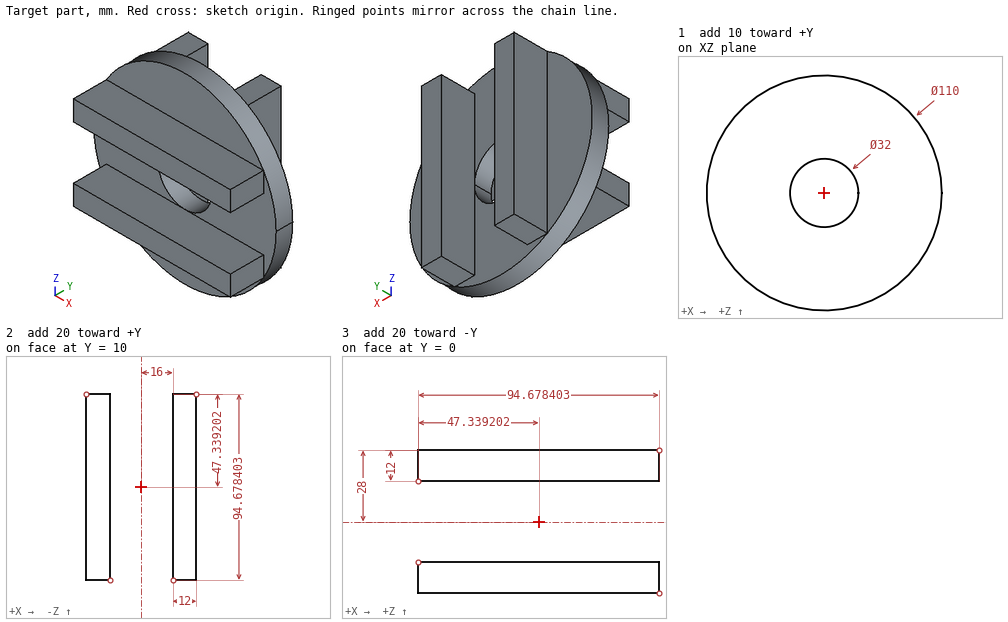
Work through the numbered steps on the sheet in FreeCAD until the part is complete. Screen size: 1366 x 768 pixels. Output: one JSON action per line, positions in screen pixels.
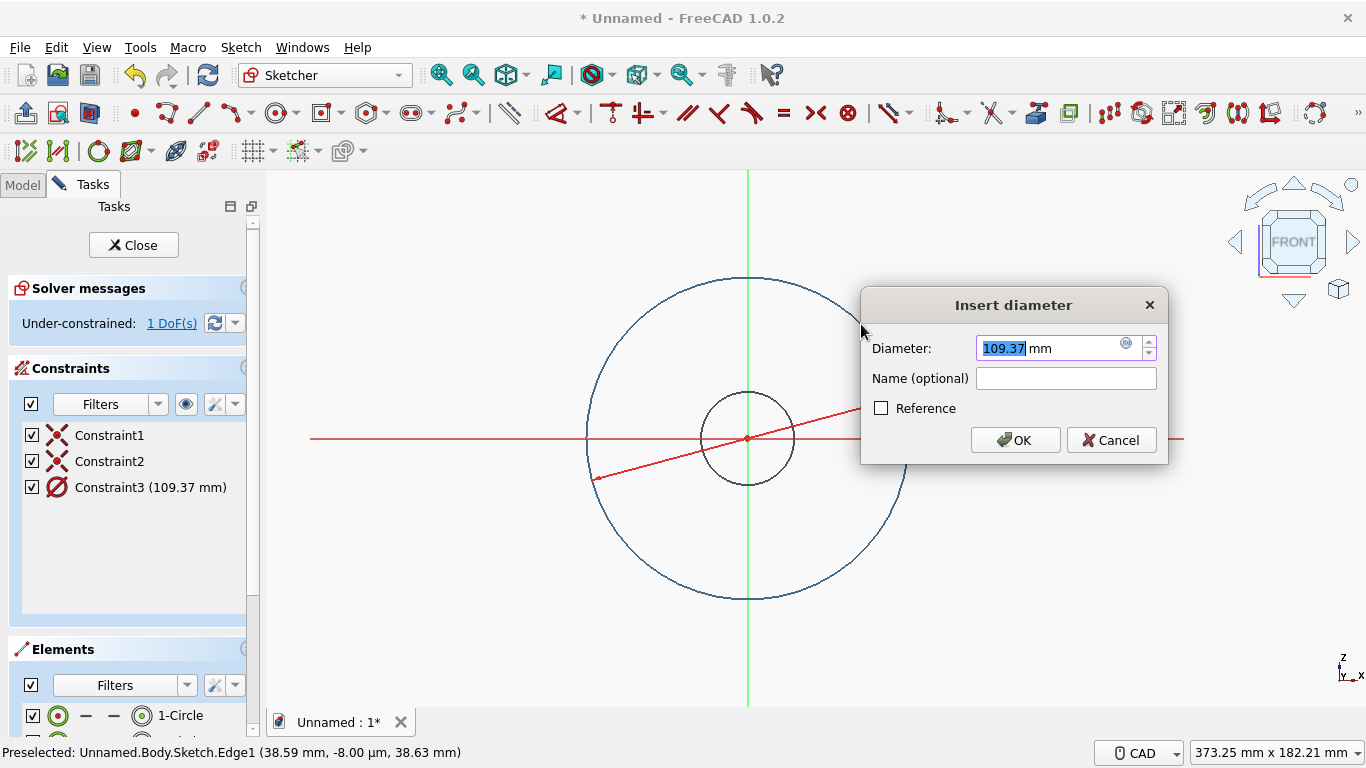
{"action": "type", "text": "110"}
{"action": "key", "text": "Return"}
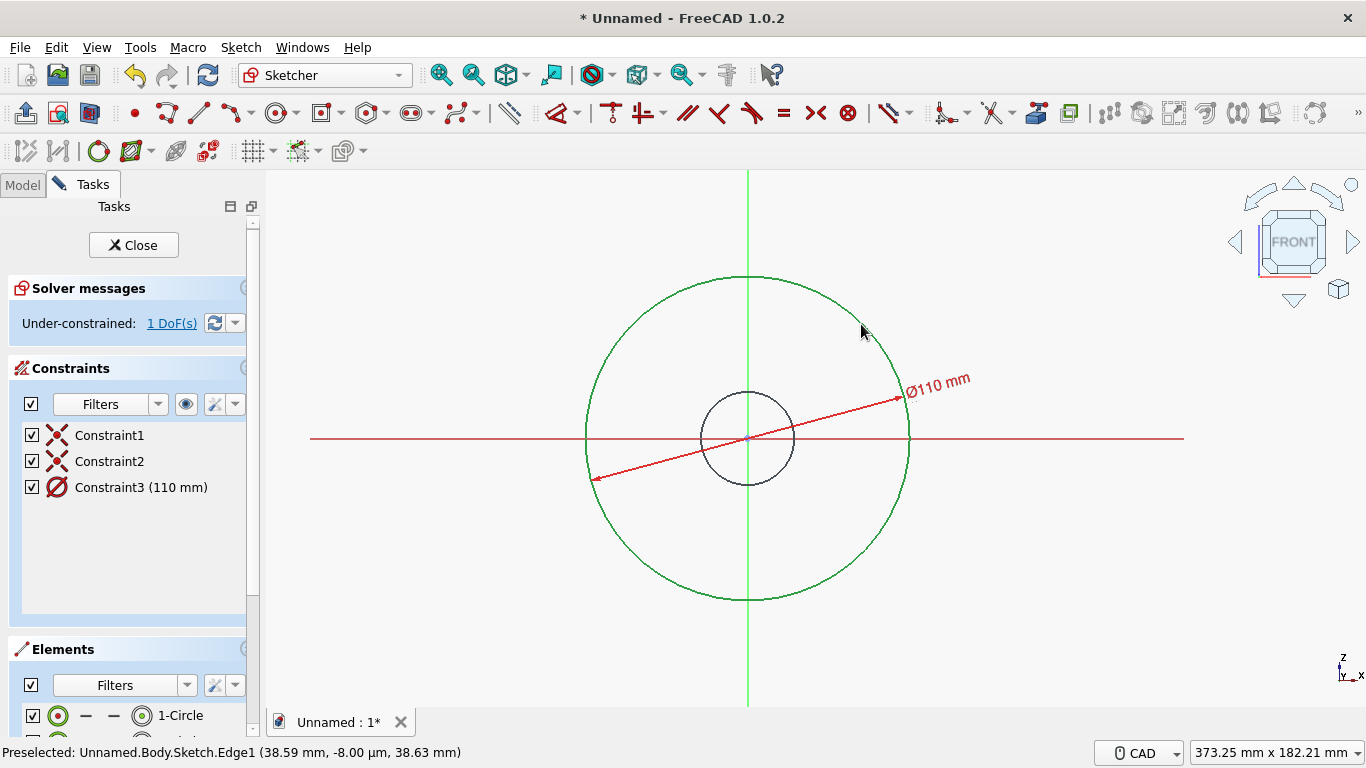
{"action": "left_click", "coordinate": [780, 405]}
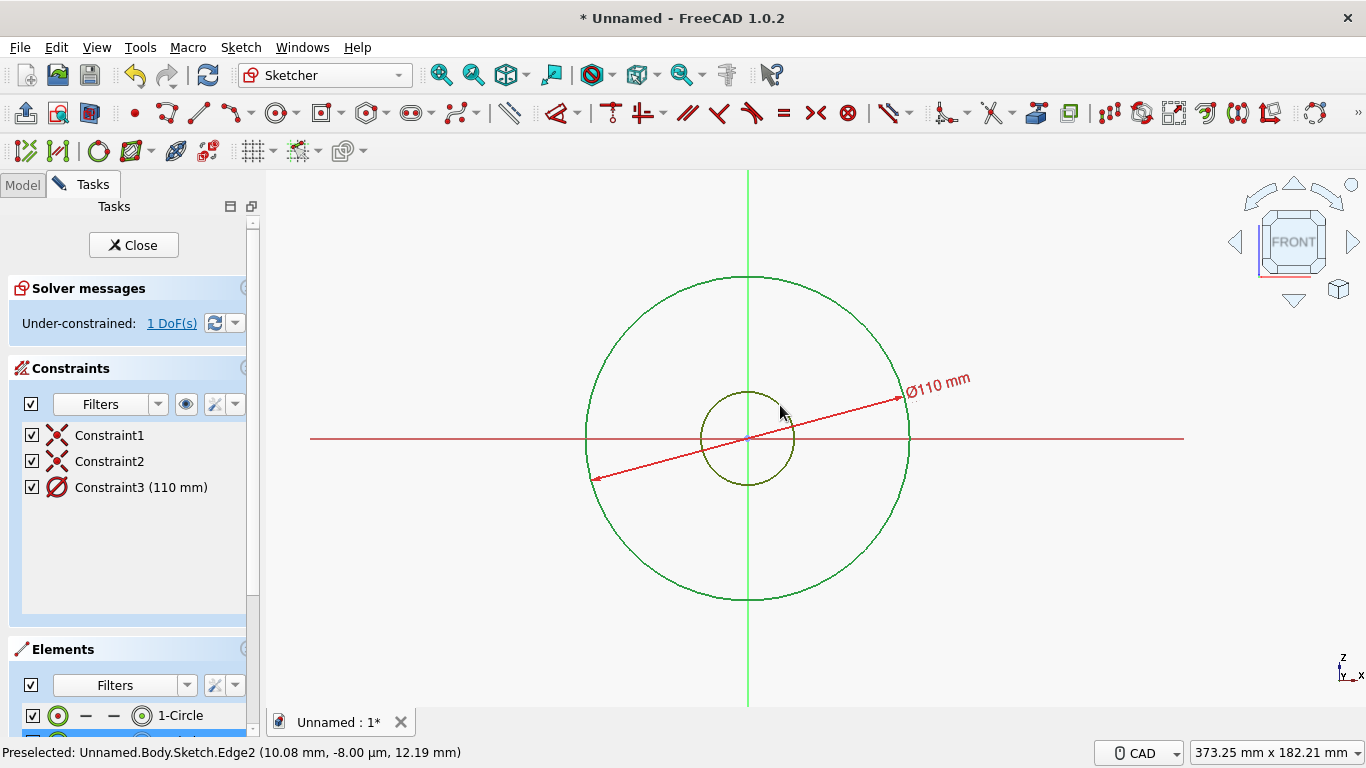
{"action": "key", "text": "k o"}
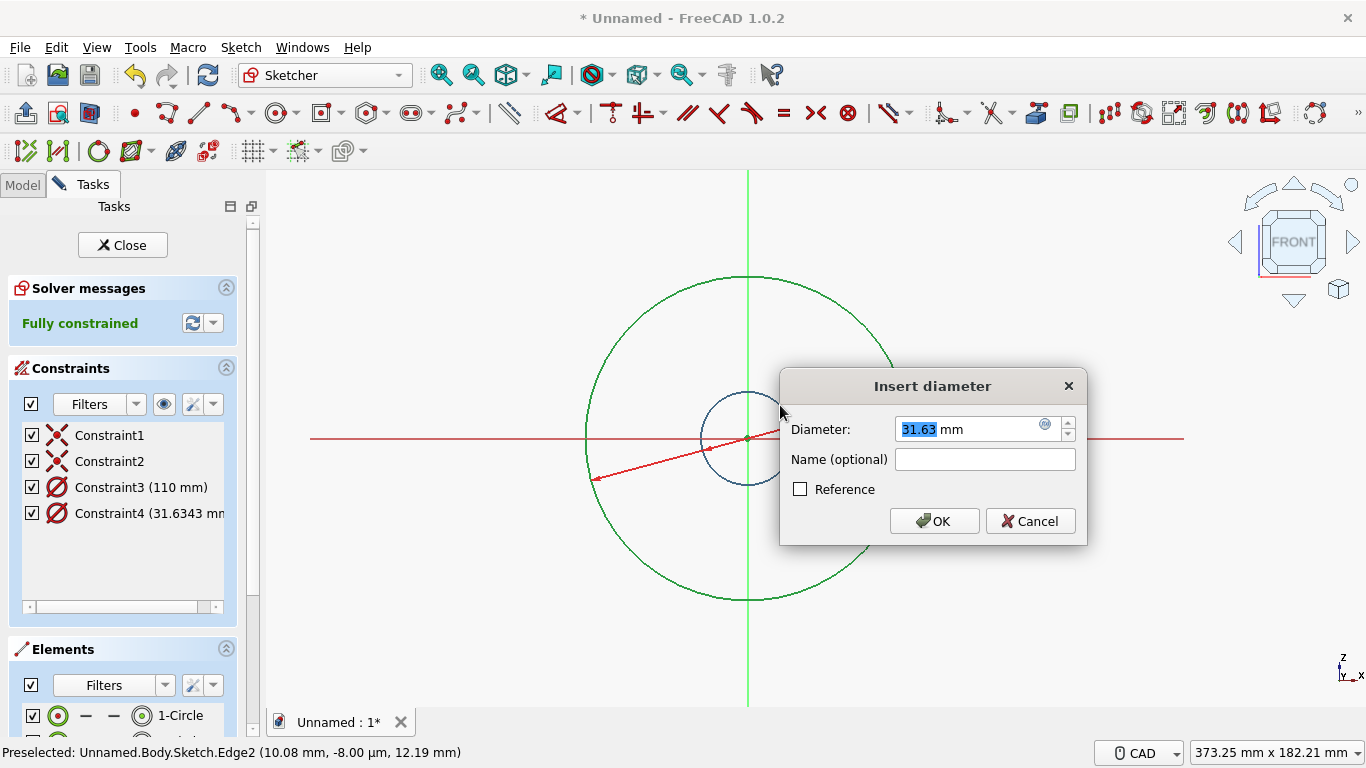
{"action": "type", "text": "32"}
{"action": "key", "text": "Return"}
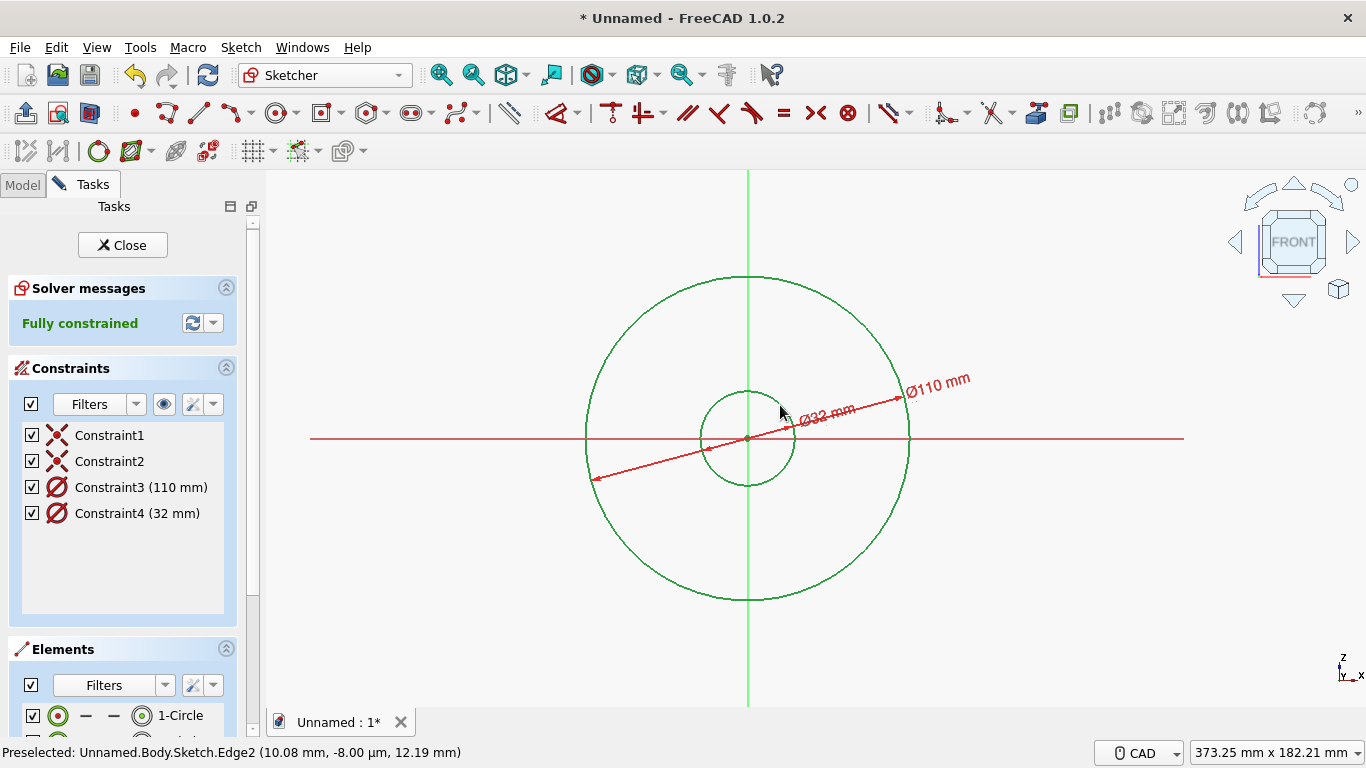
{"action": "left_click", "coordinate": [123, 245]}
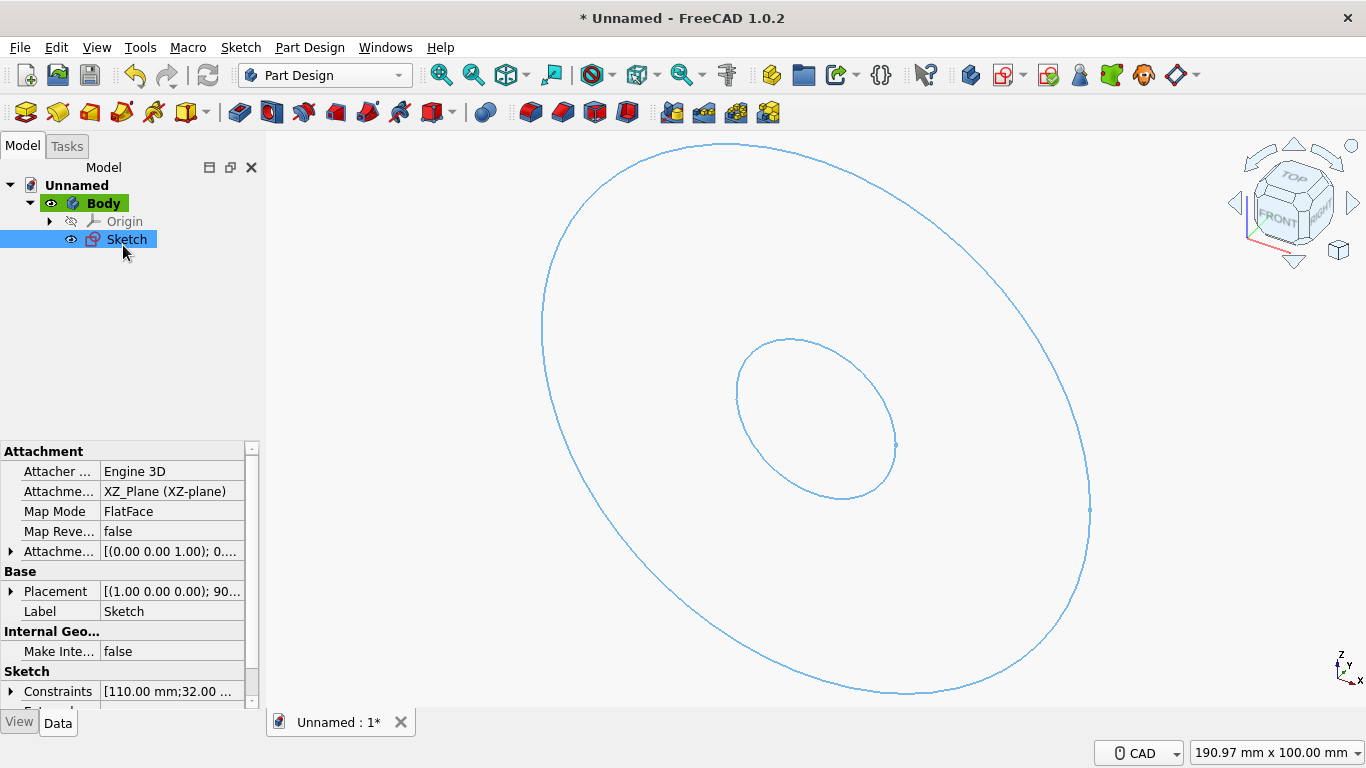
{"action": "left_click", "coordinate": [26, 112]}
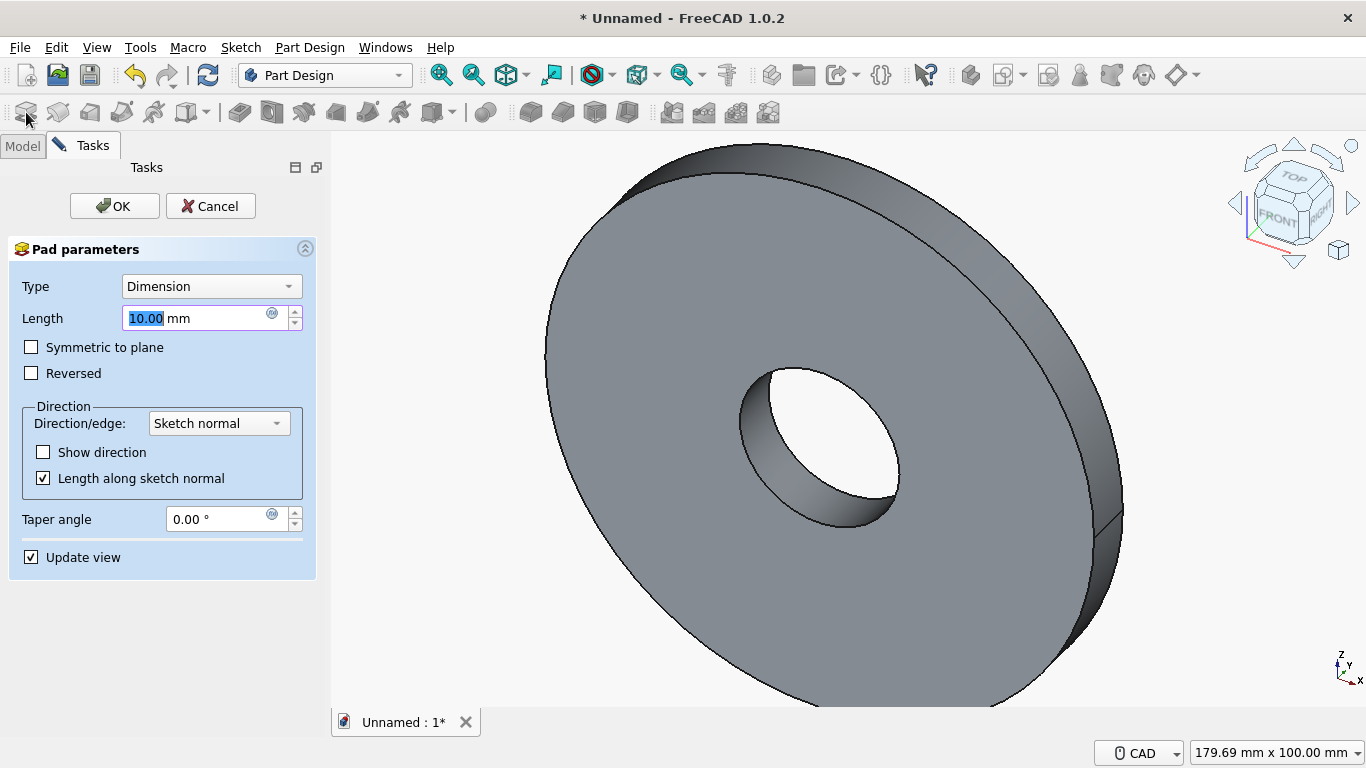
{"action": "type", "text": "10"}
{"action": "key", "text": "Tab"}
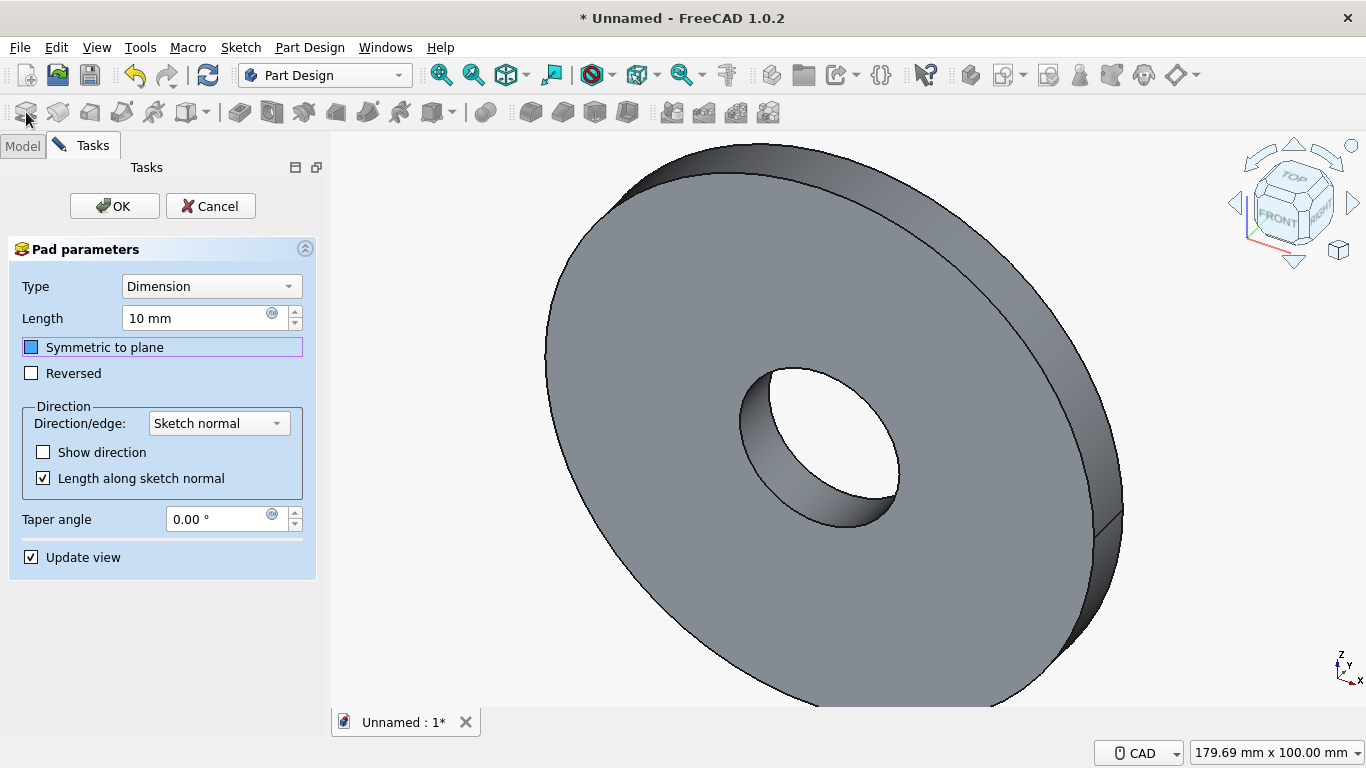
{"action": "left_click", "coordinate": [30, 373]}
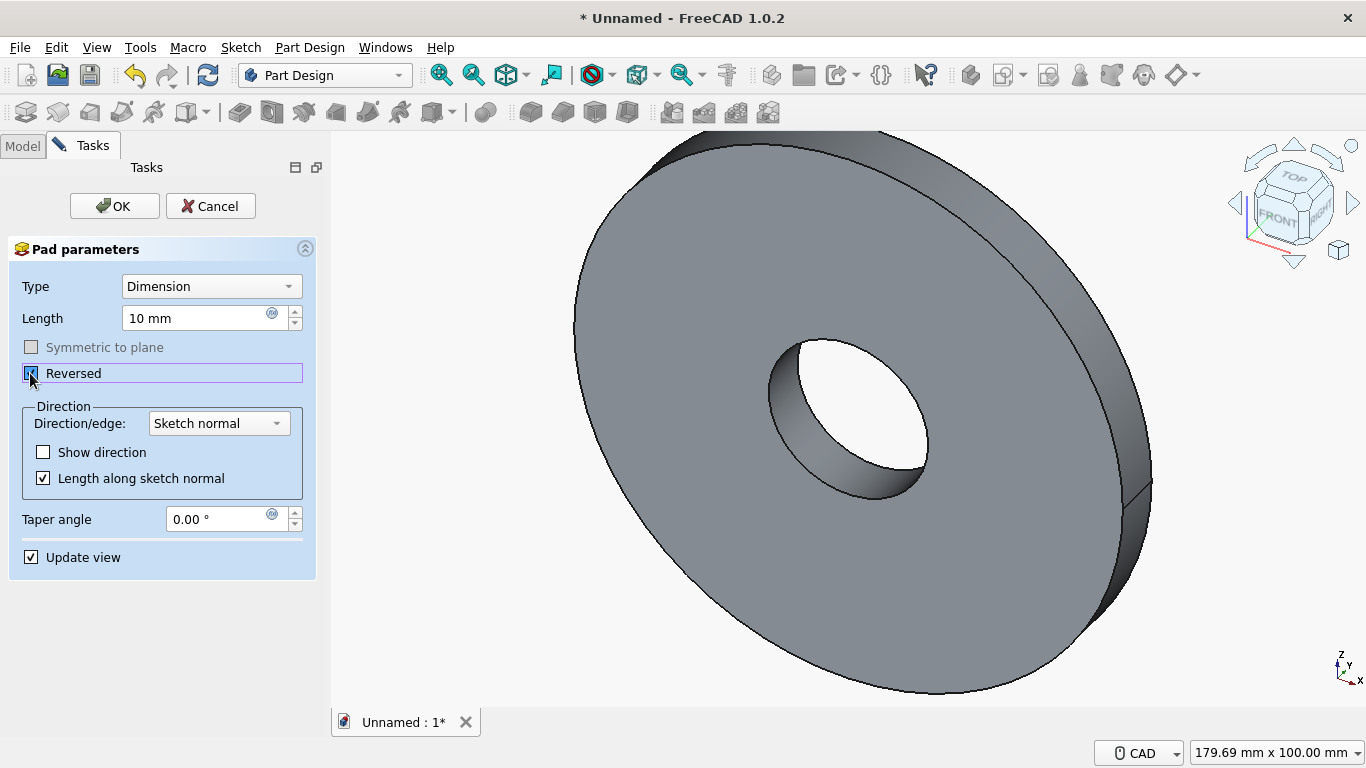
{"action": "left_click", "coordinate": [115, 206]}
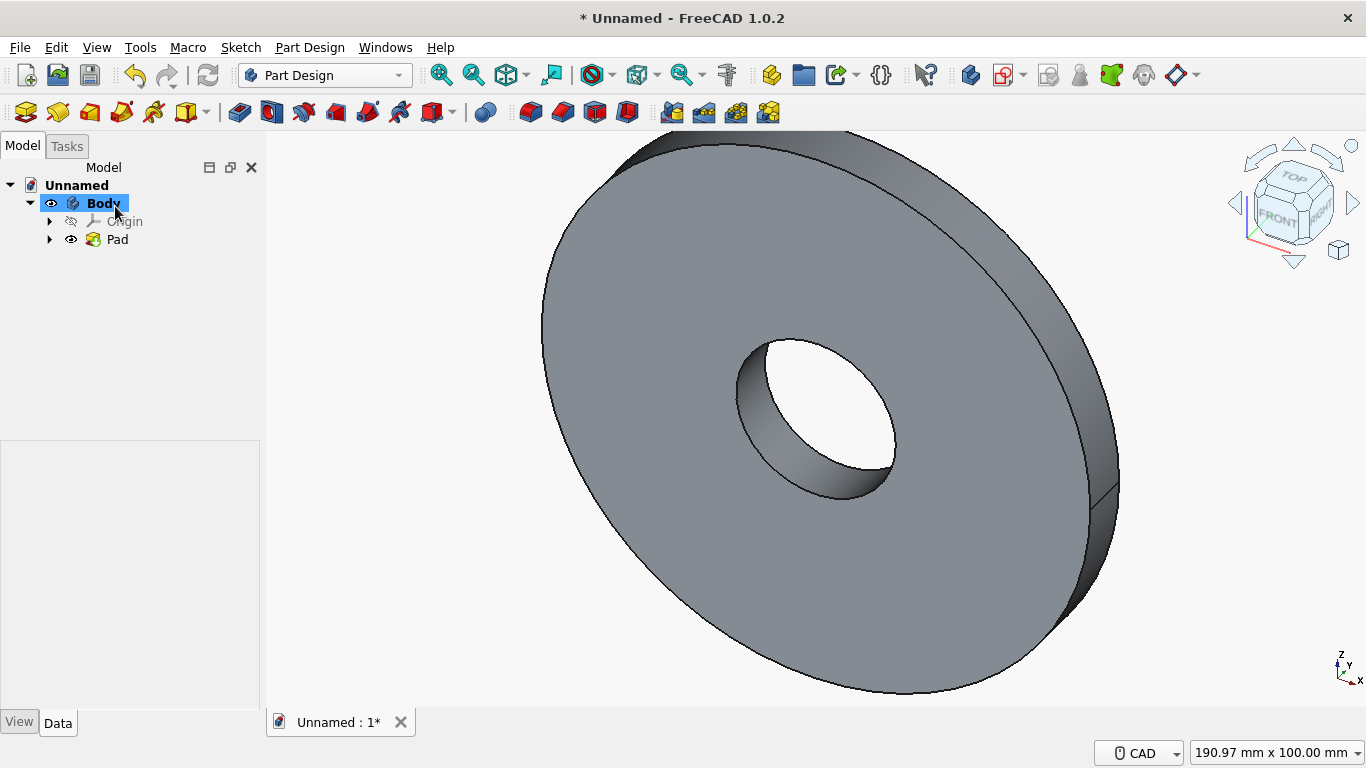
{"action": "left_click", "coordinate": [442, 76]}